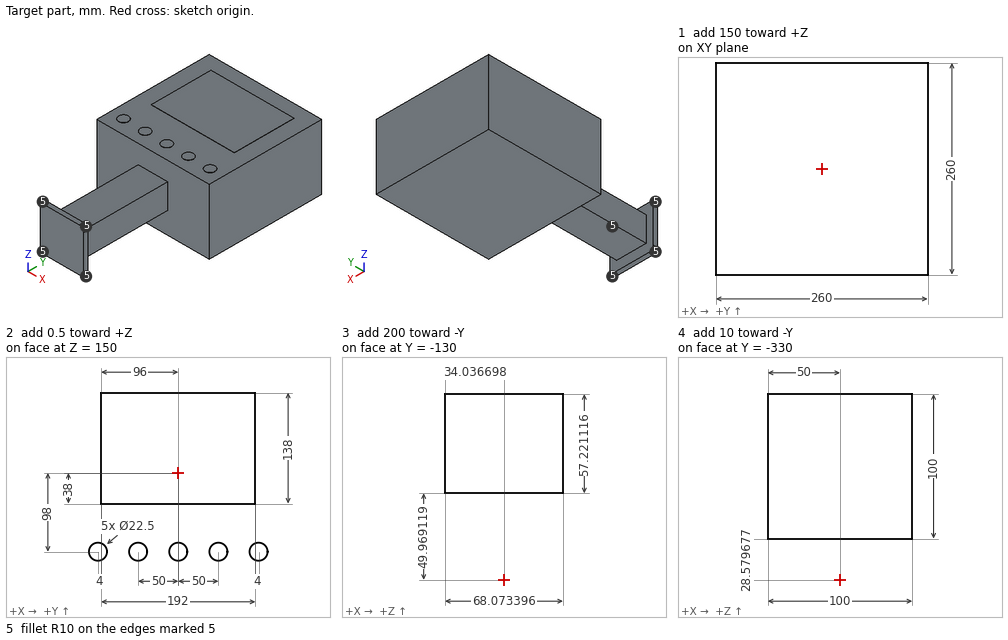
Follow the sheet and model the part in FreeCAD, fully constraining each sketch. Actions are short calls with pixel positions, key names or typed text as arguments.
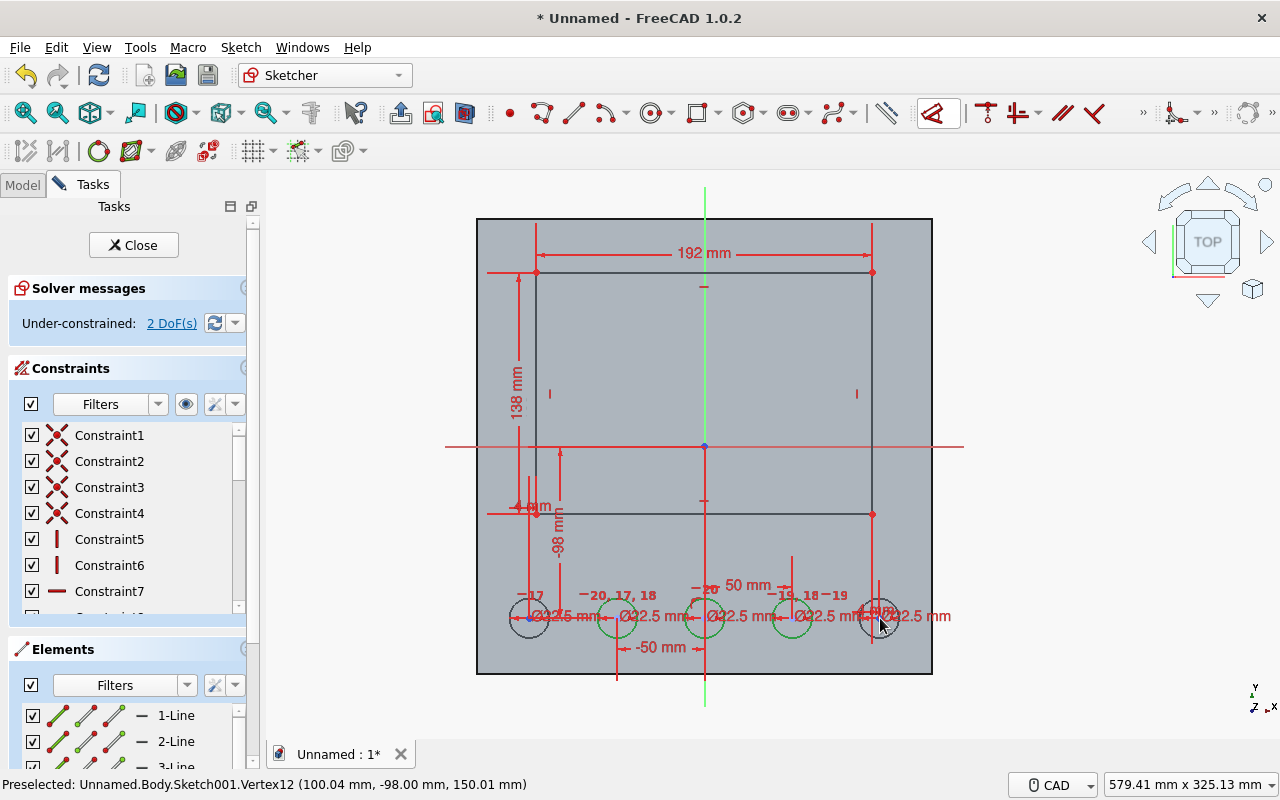
click(536, 273)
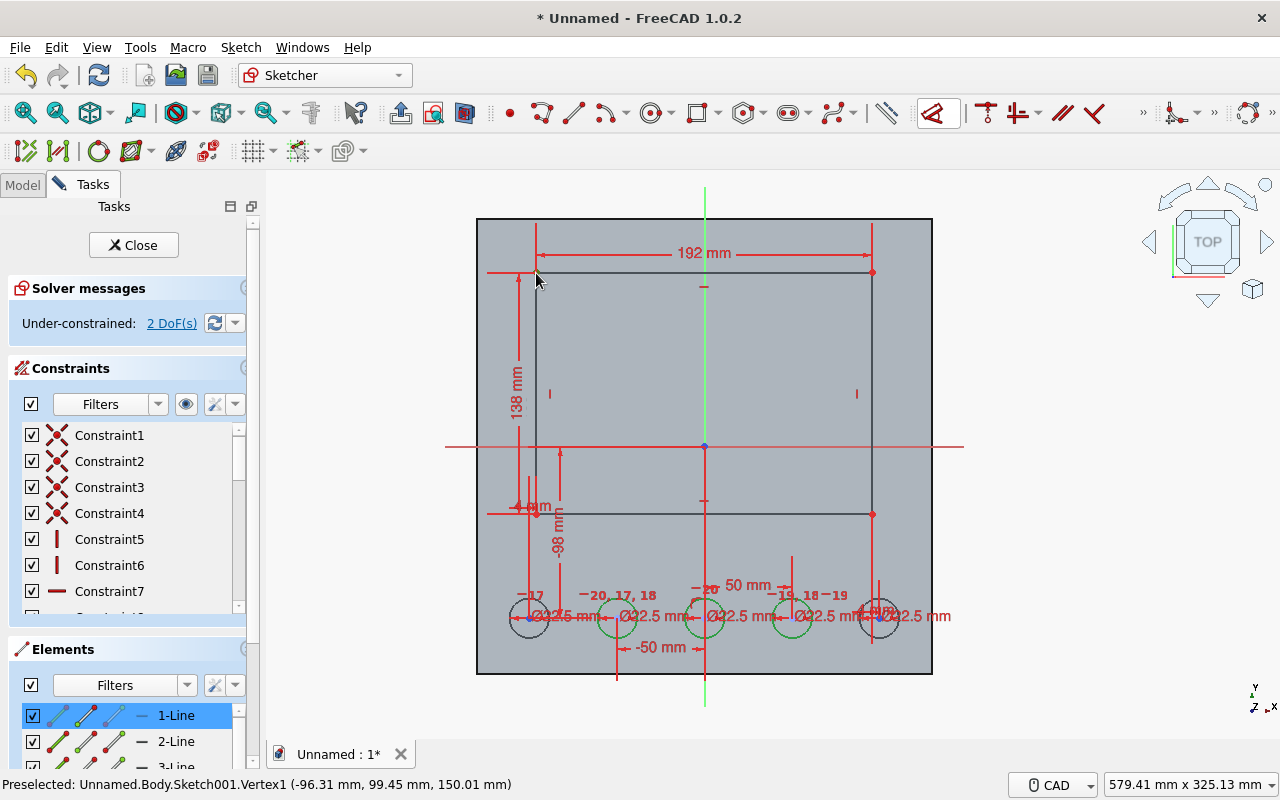
key(l)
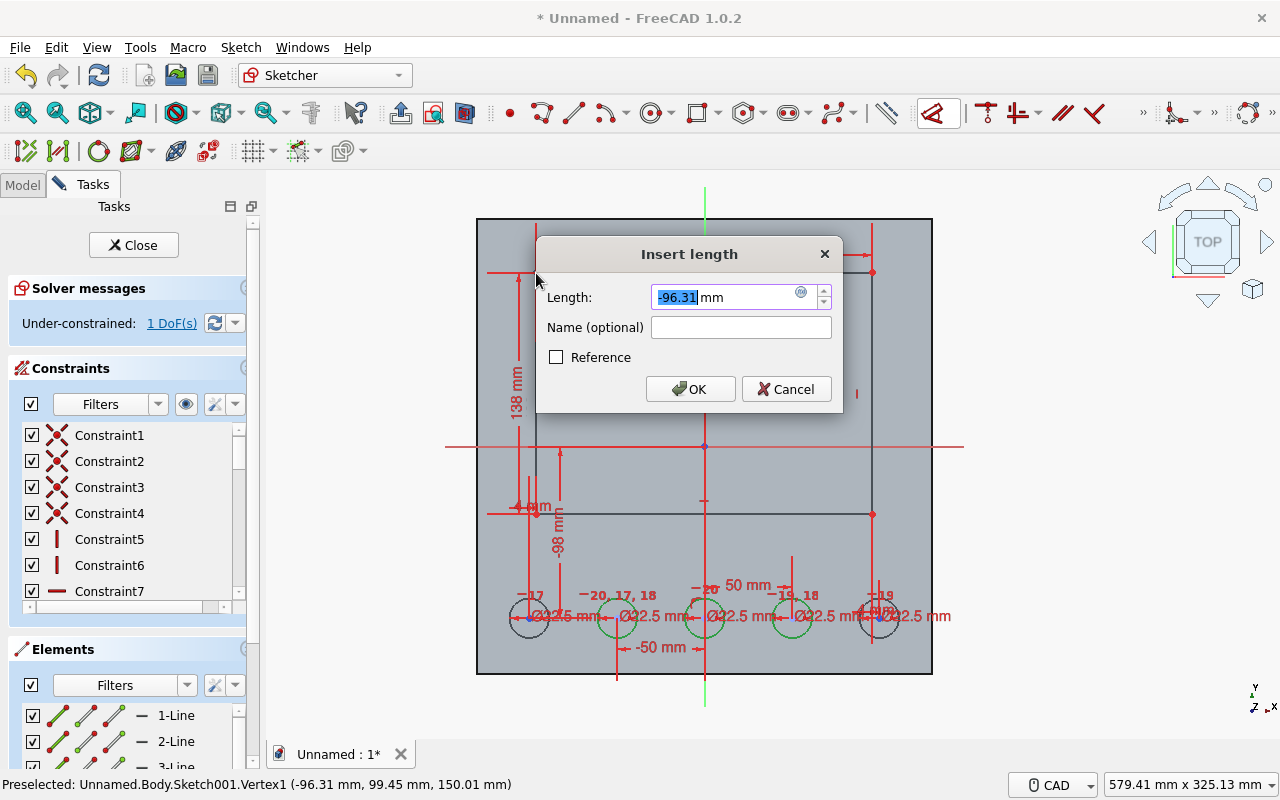
text(-96)
key(Return)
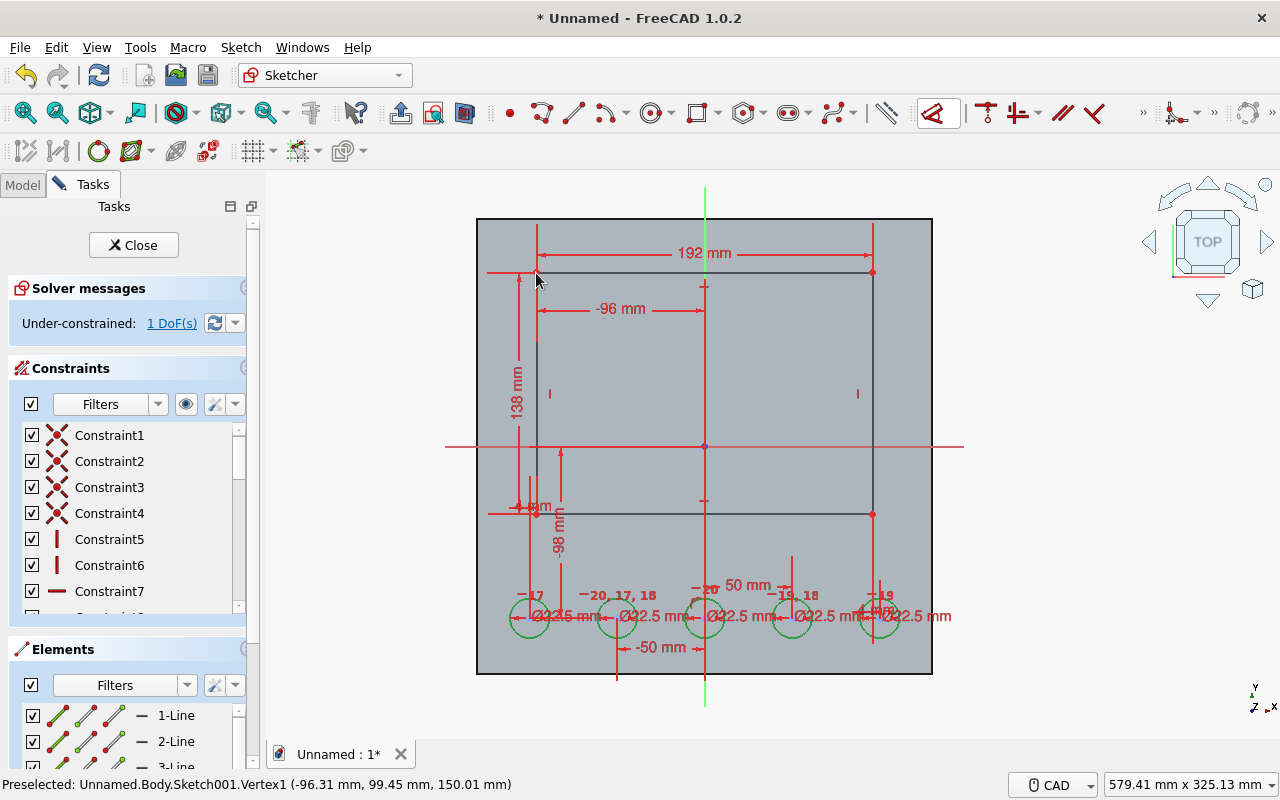
click(537, 514)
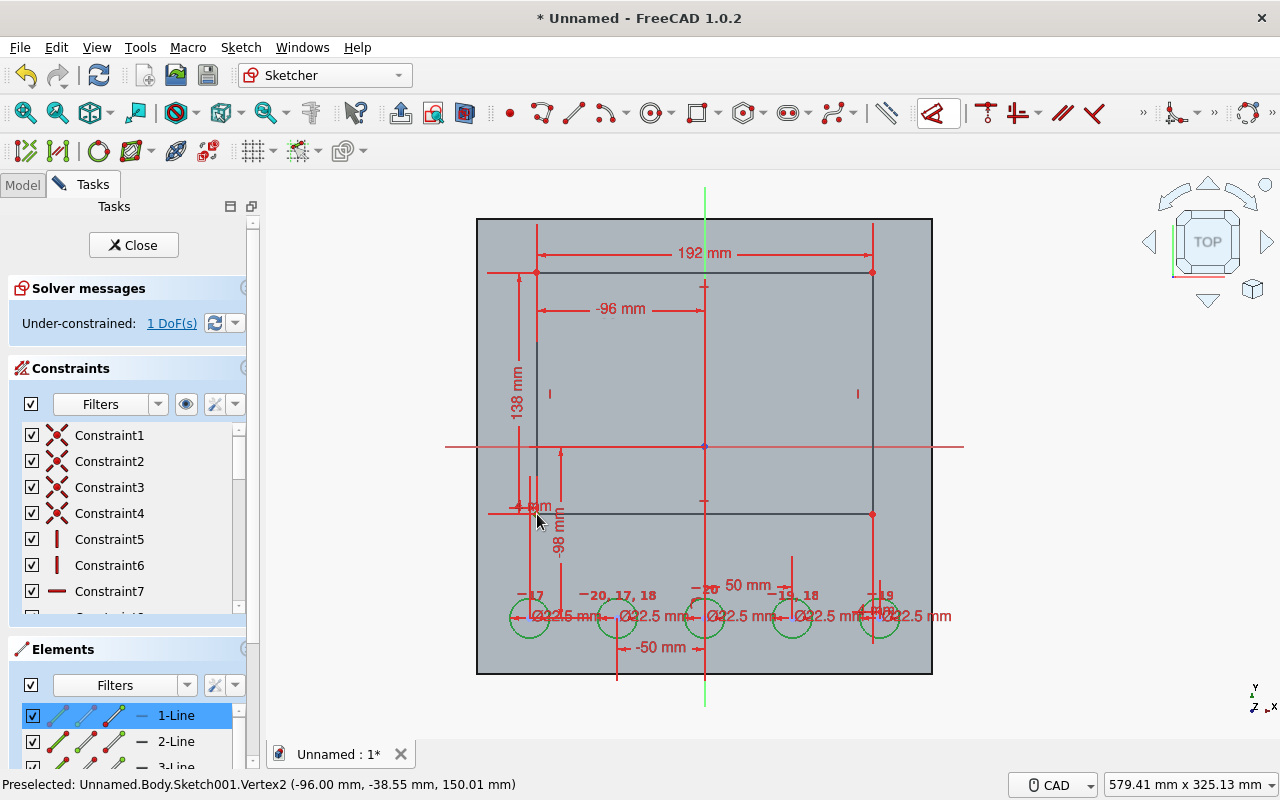
click(954, 114)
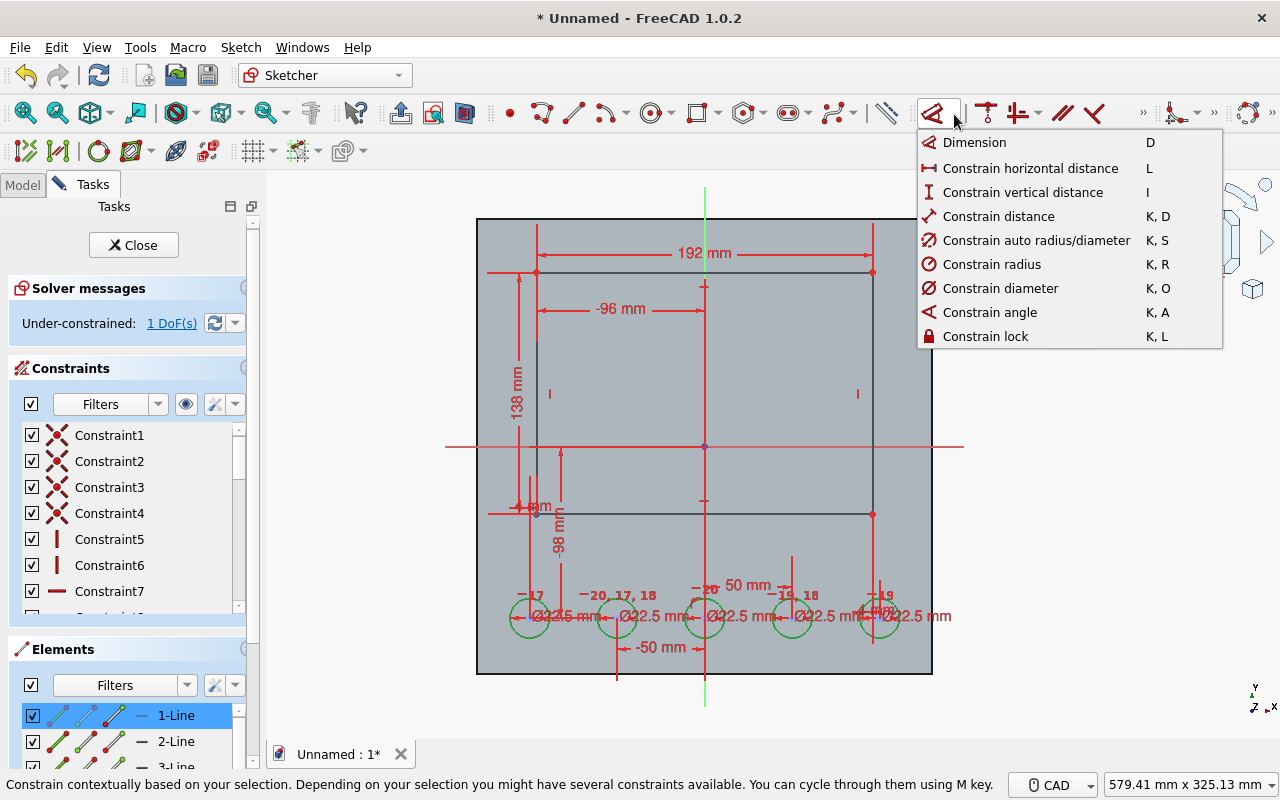
click(1070, 192)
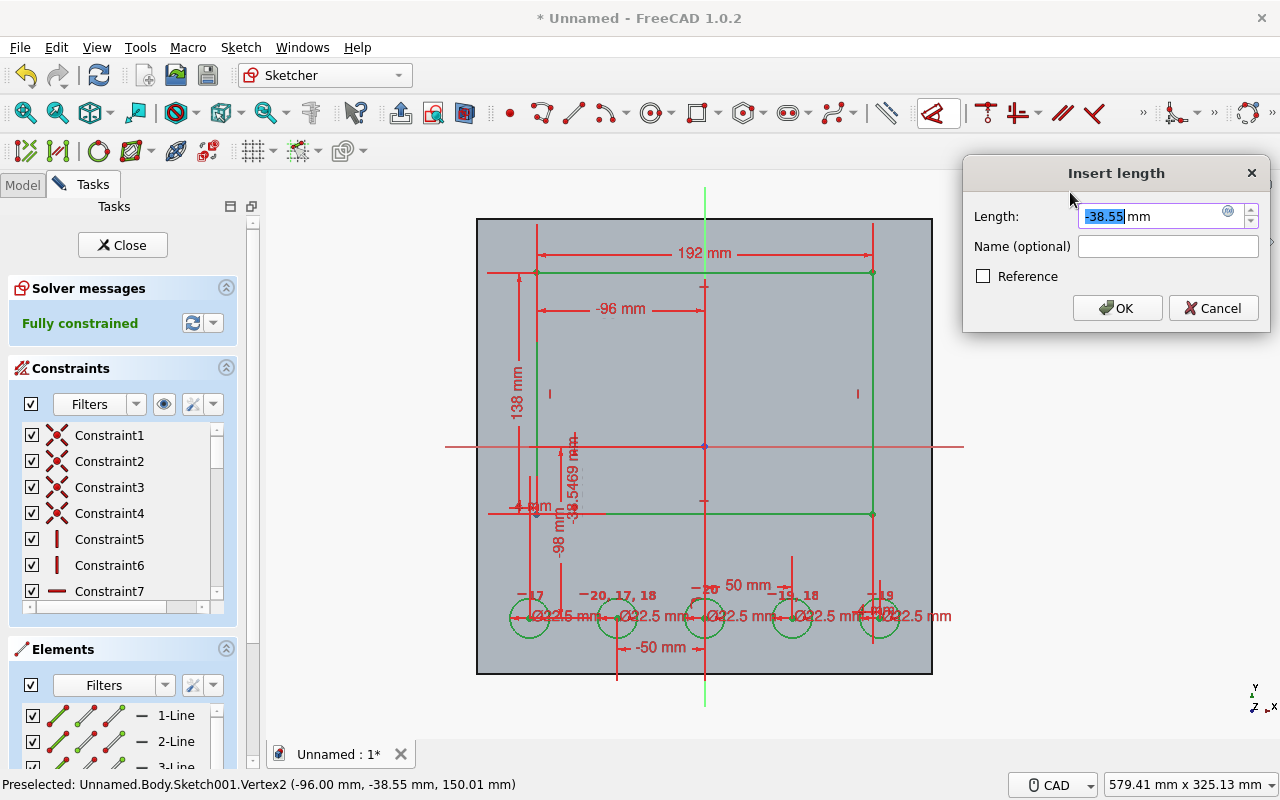
text(-38)
key(Return)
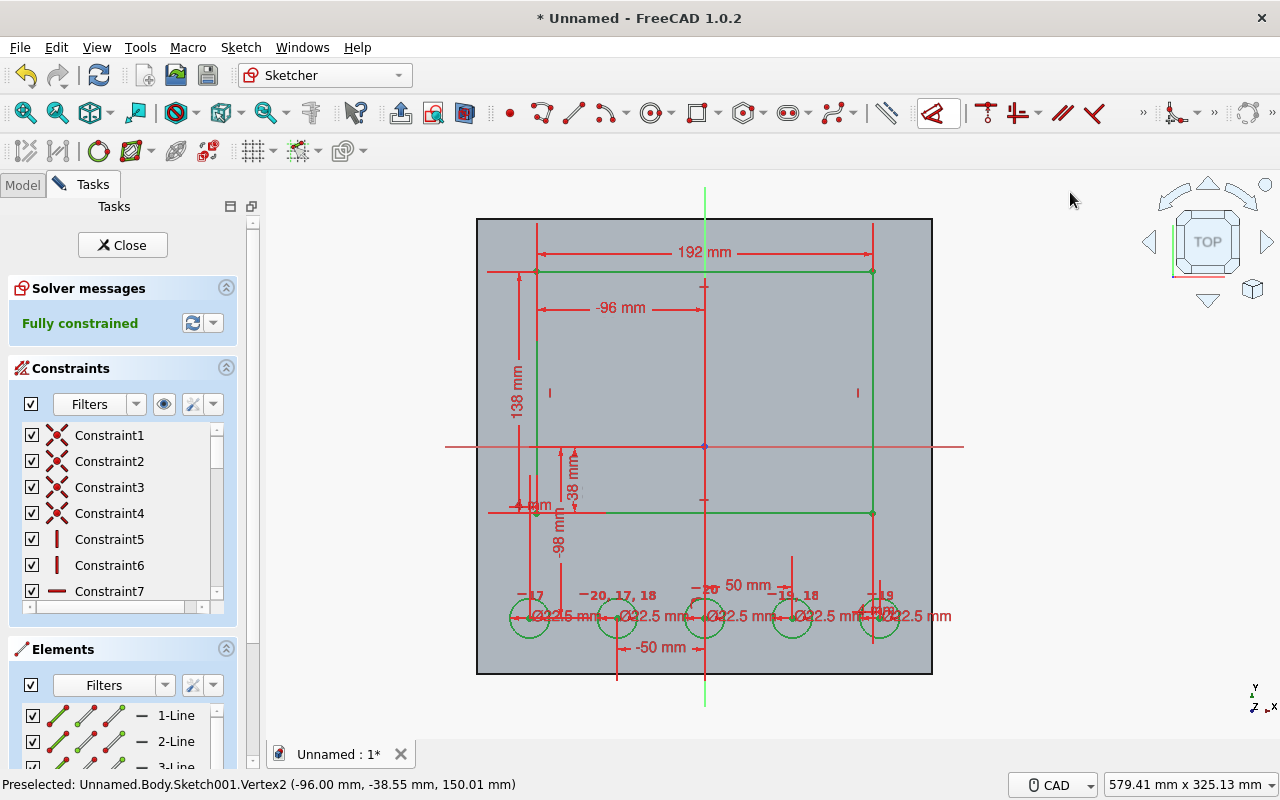
click(123, 245)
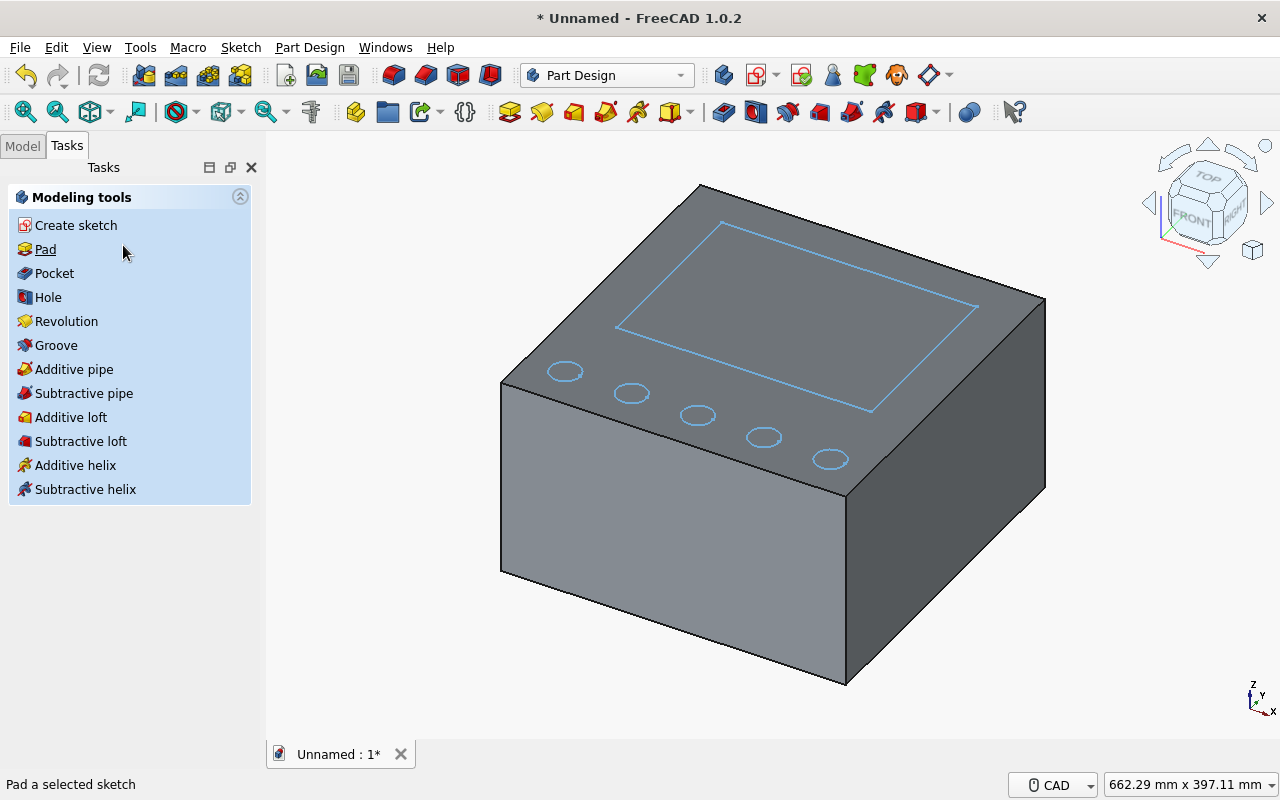
click(510, 112)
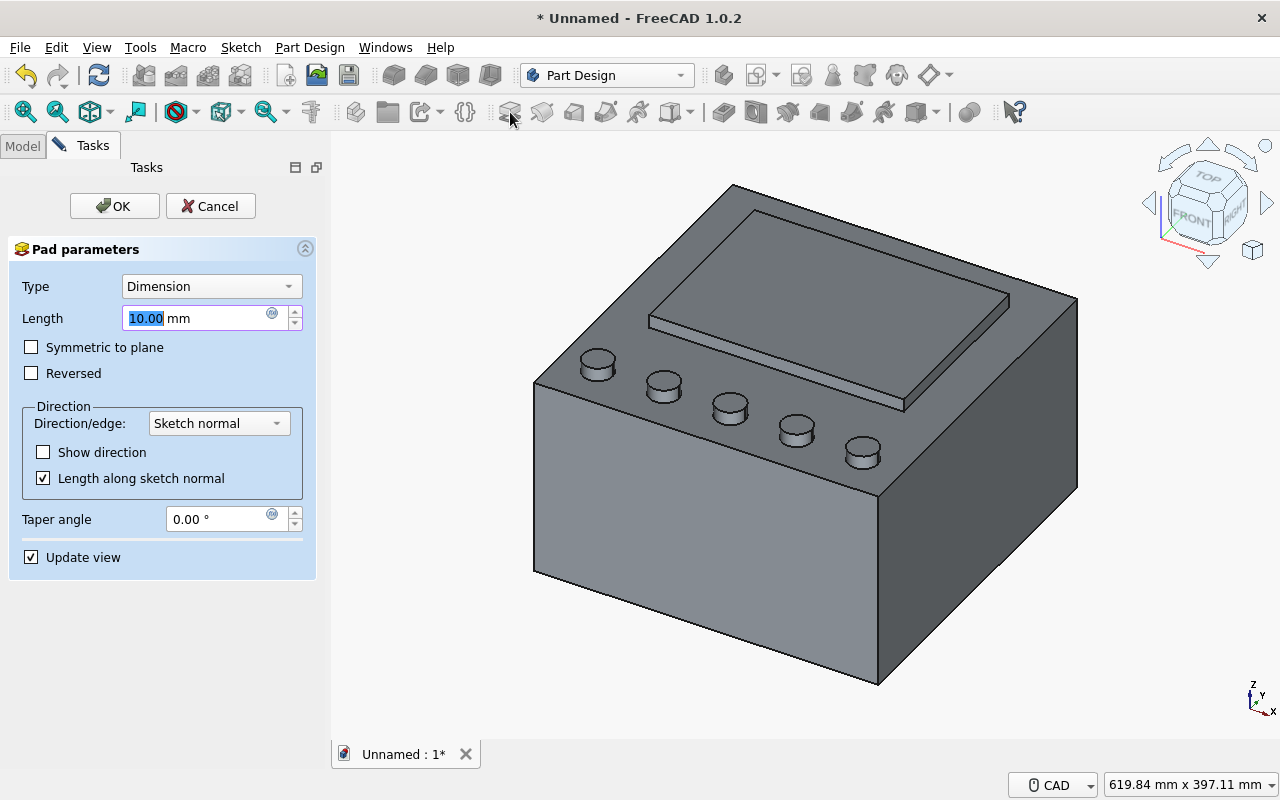
text(0.5)
key(Tab)